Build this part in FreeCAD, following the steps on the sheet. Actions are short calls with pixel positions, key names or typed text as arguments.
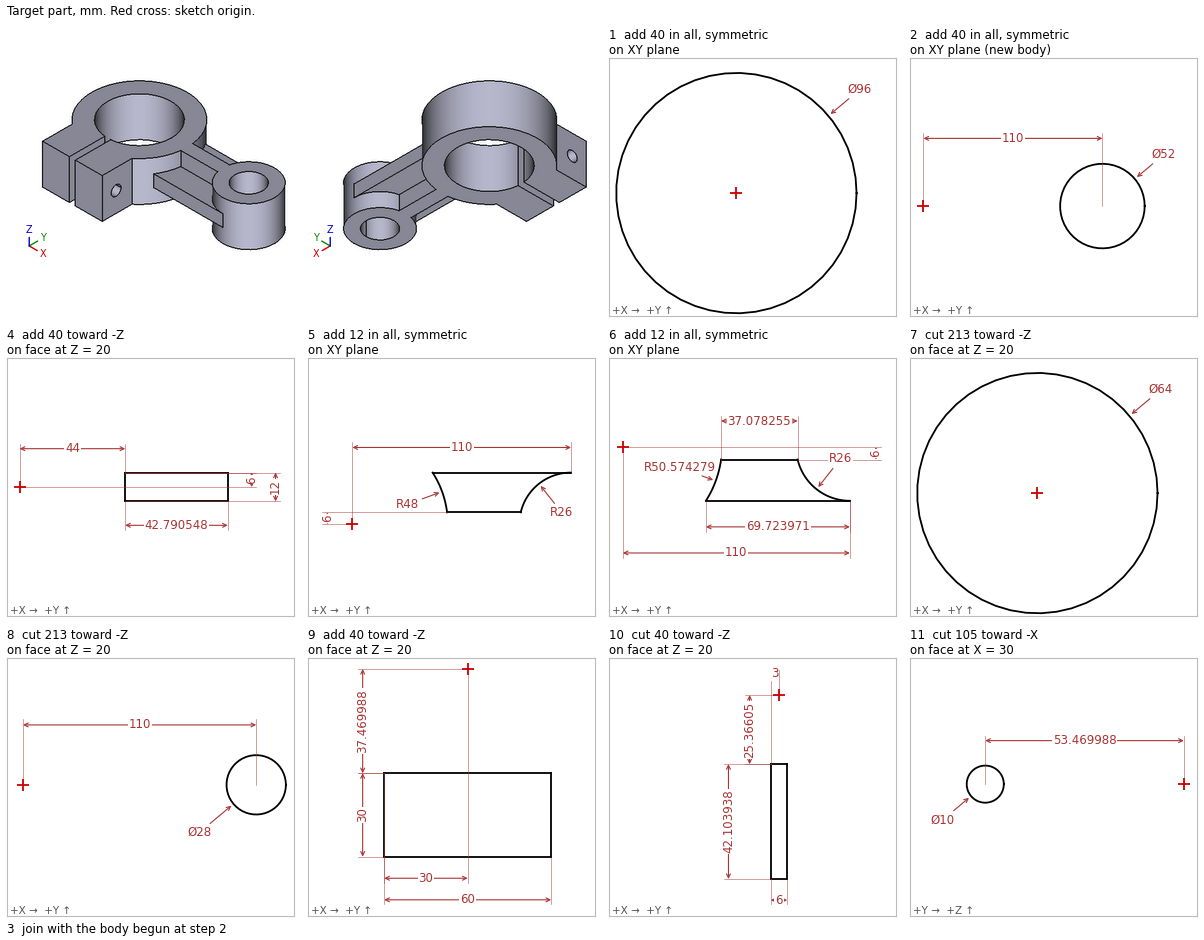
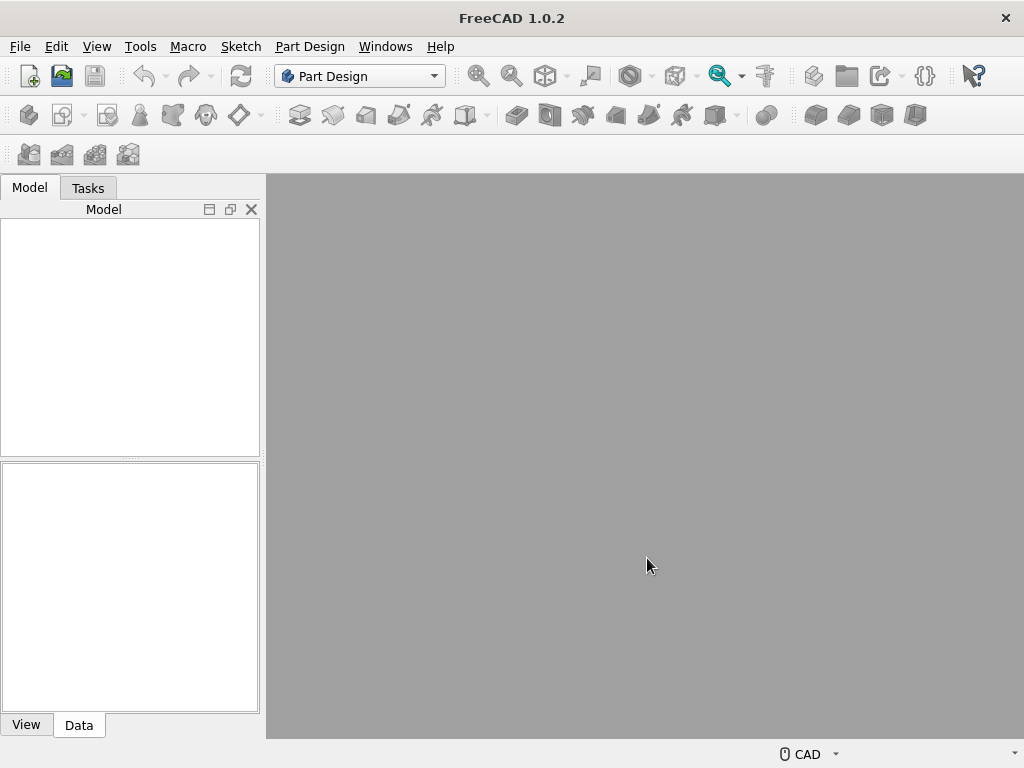
click(29, 76)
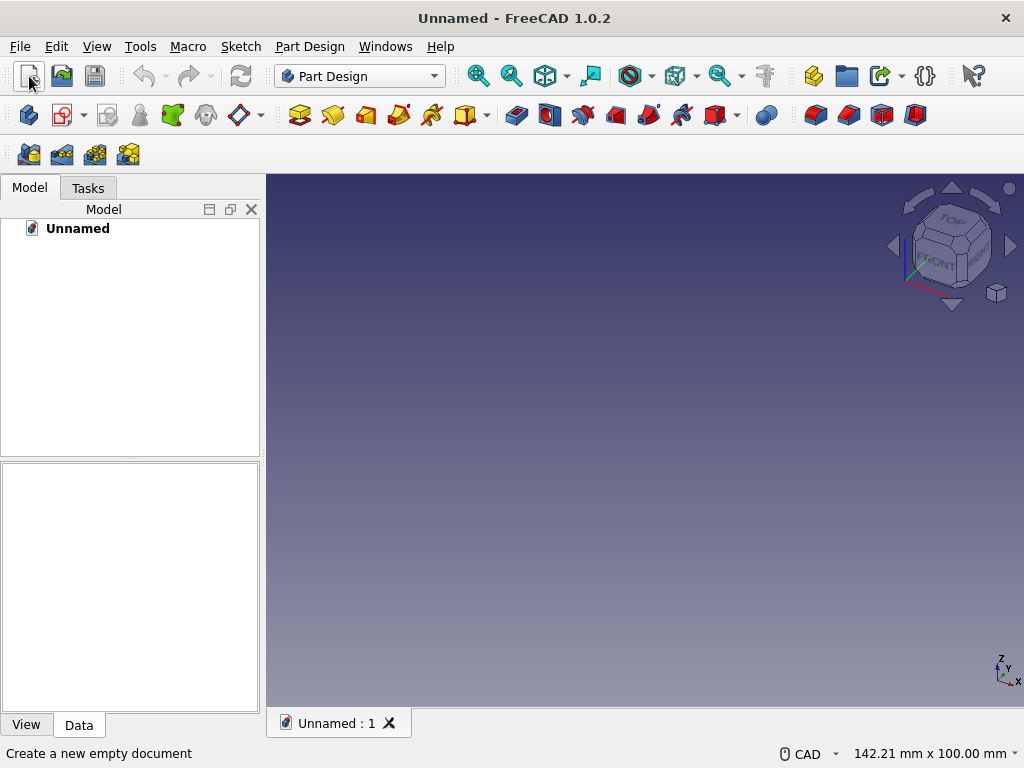
click(62, 116)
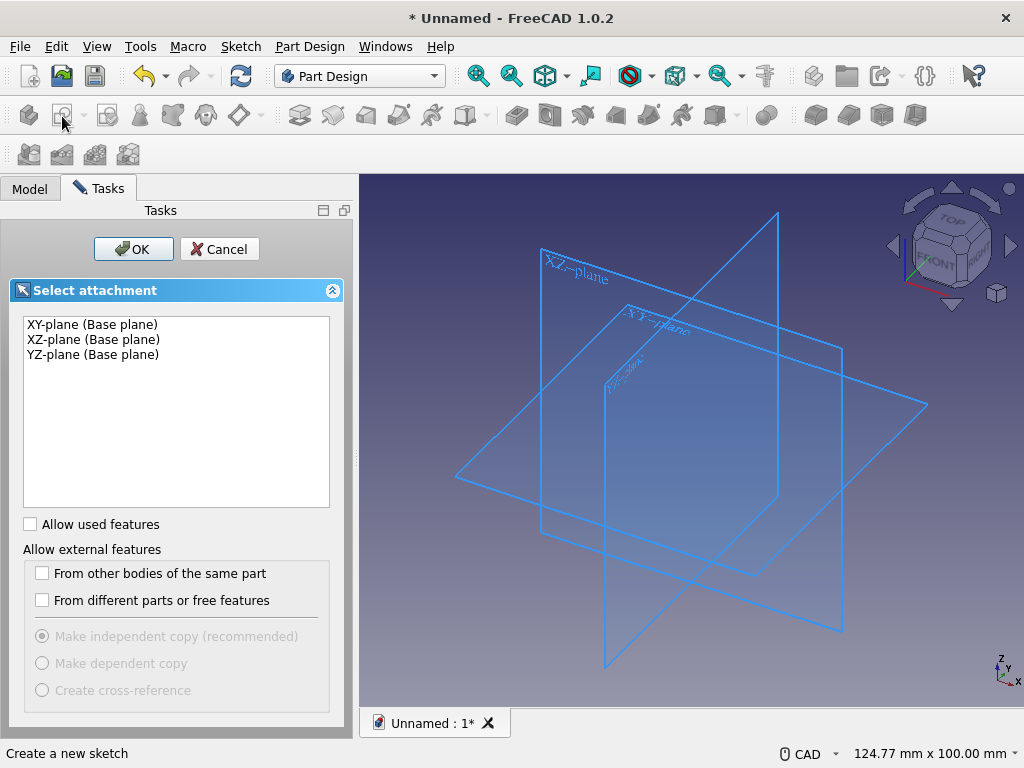
click(84, 324)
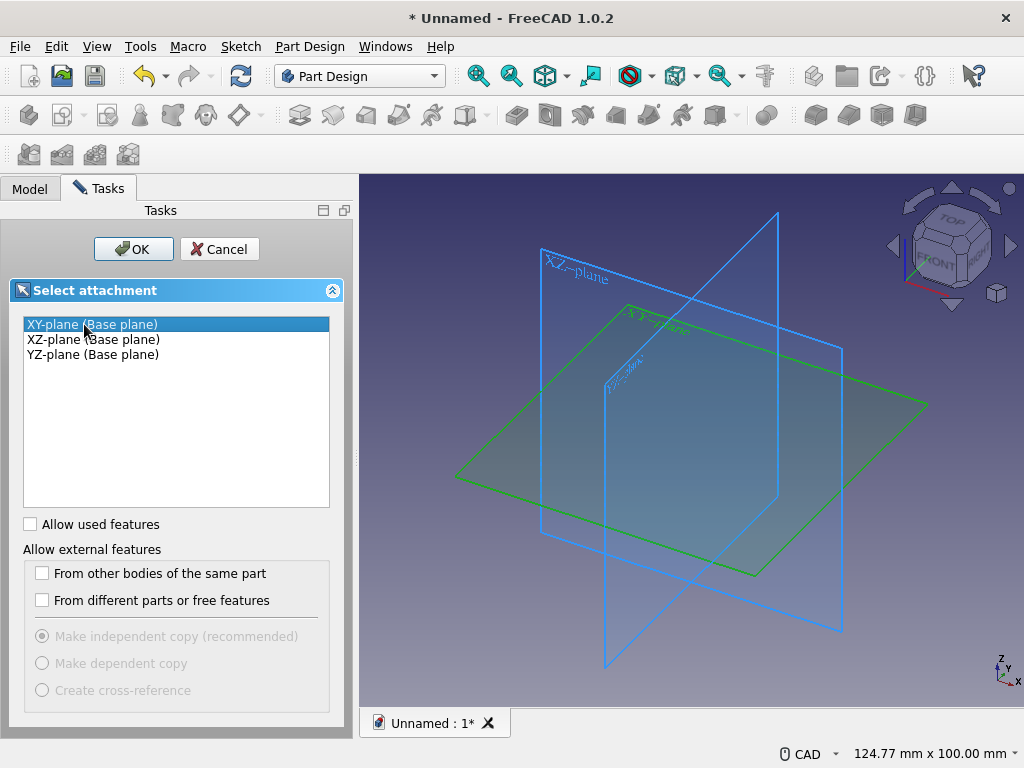
click(134, 249)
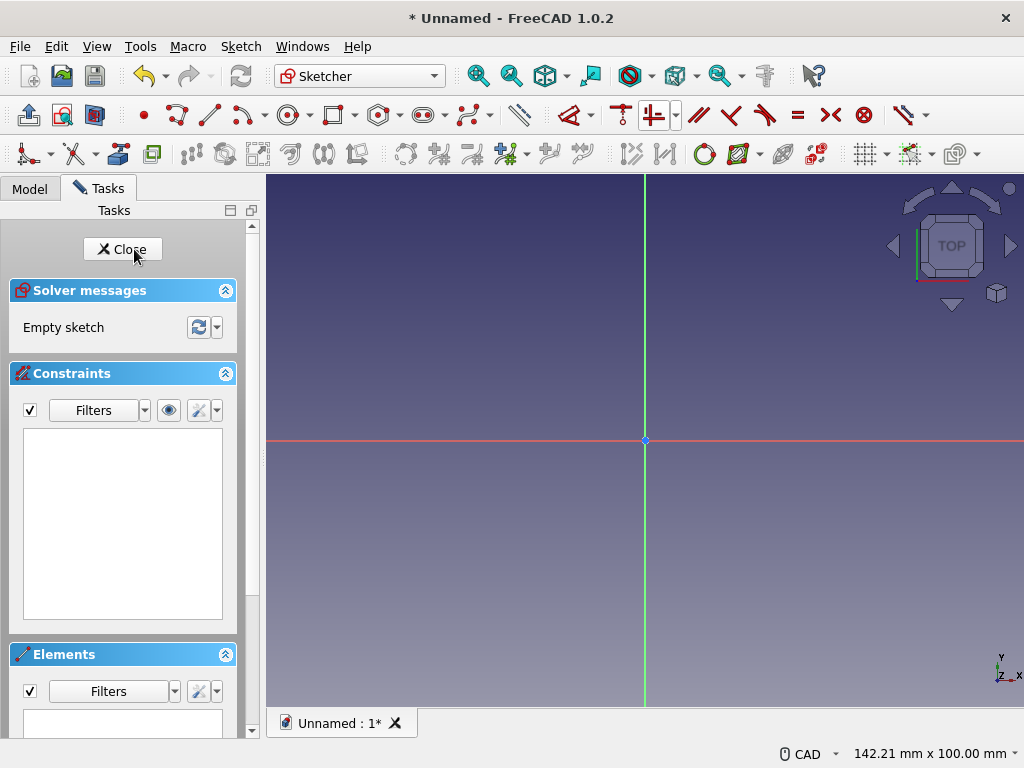
scroll(437, 440, down, 2)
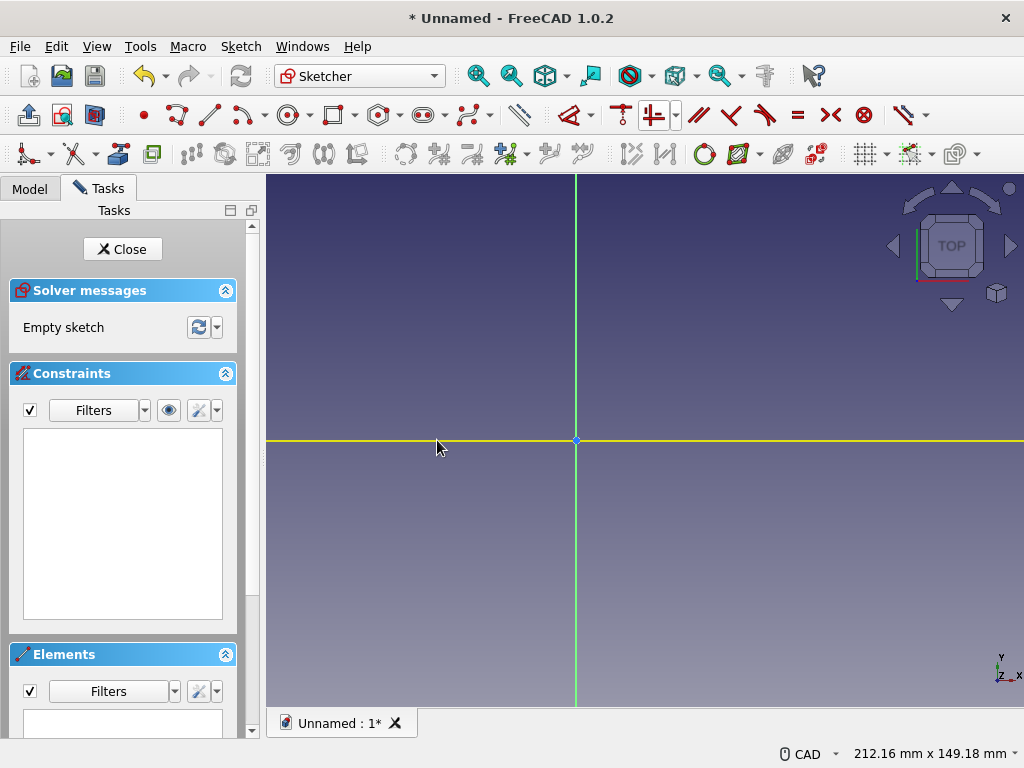
click(288, 116)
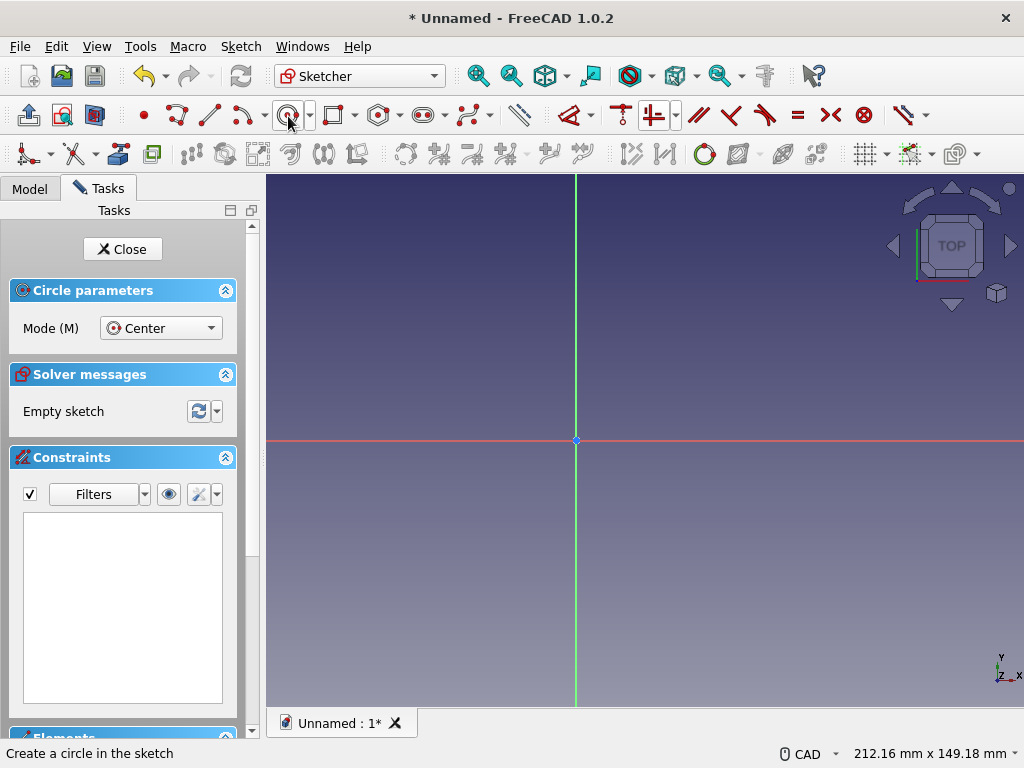
click(577, 440)
click(698, 319)
key(Escape)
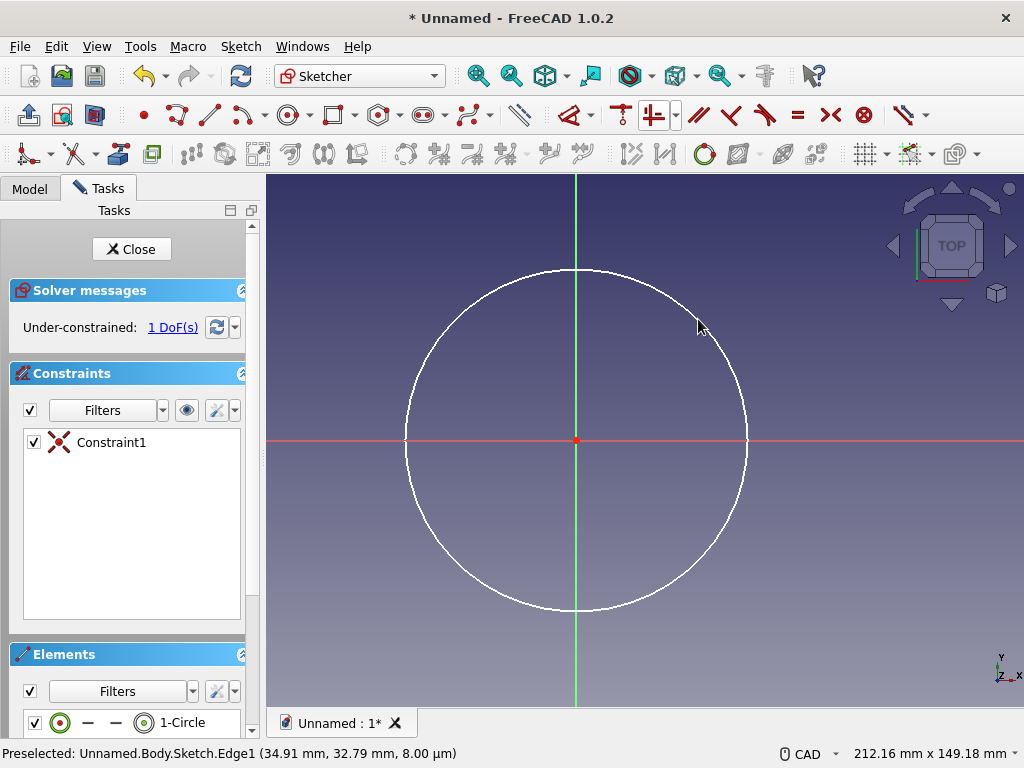
click(697, 319)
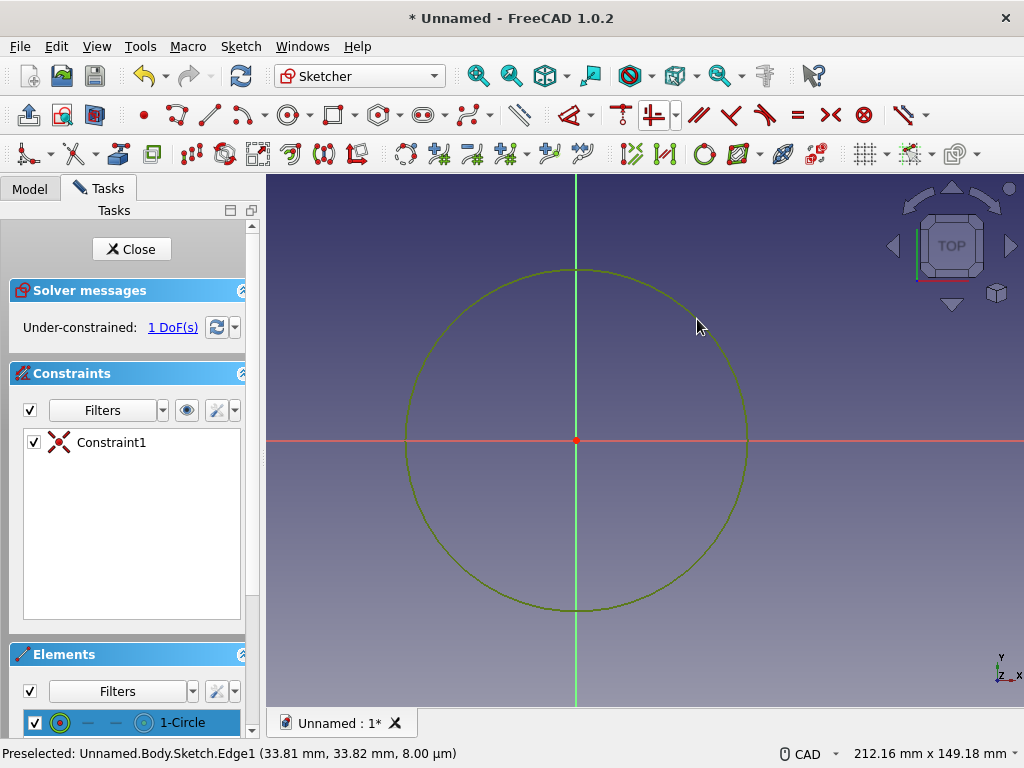
click(590, 116)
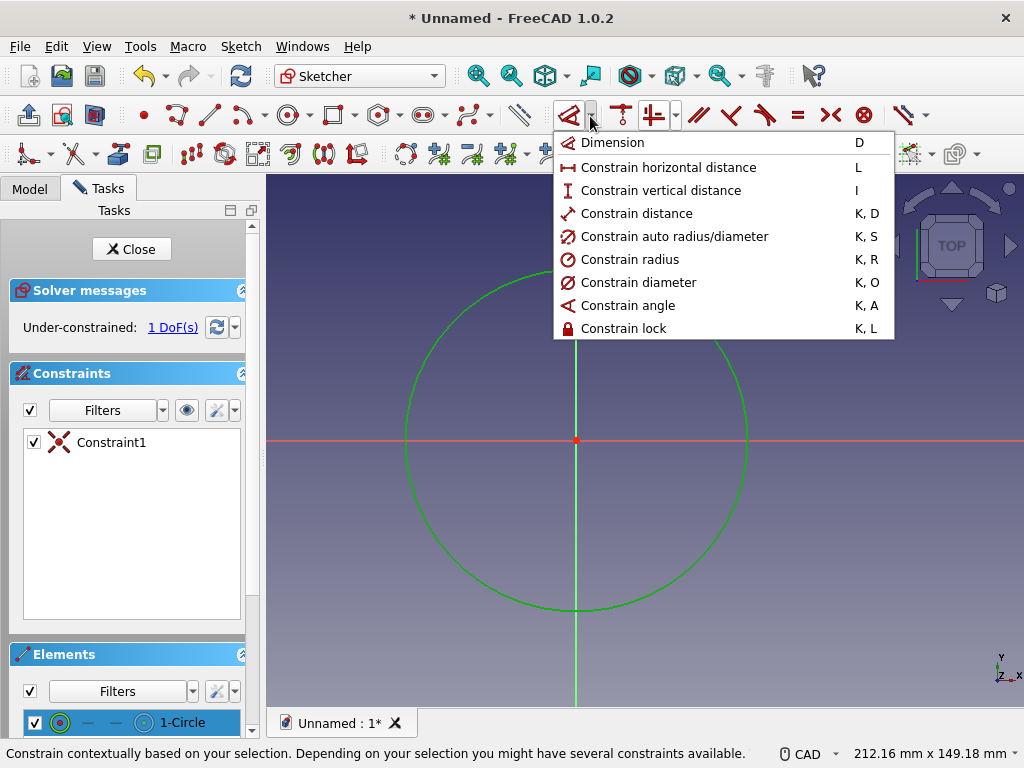
click(724, 282)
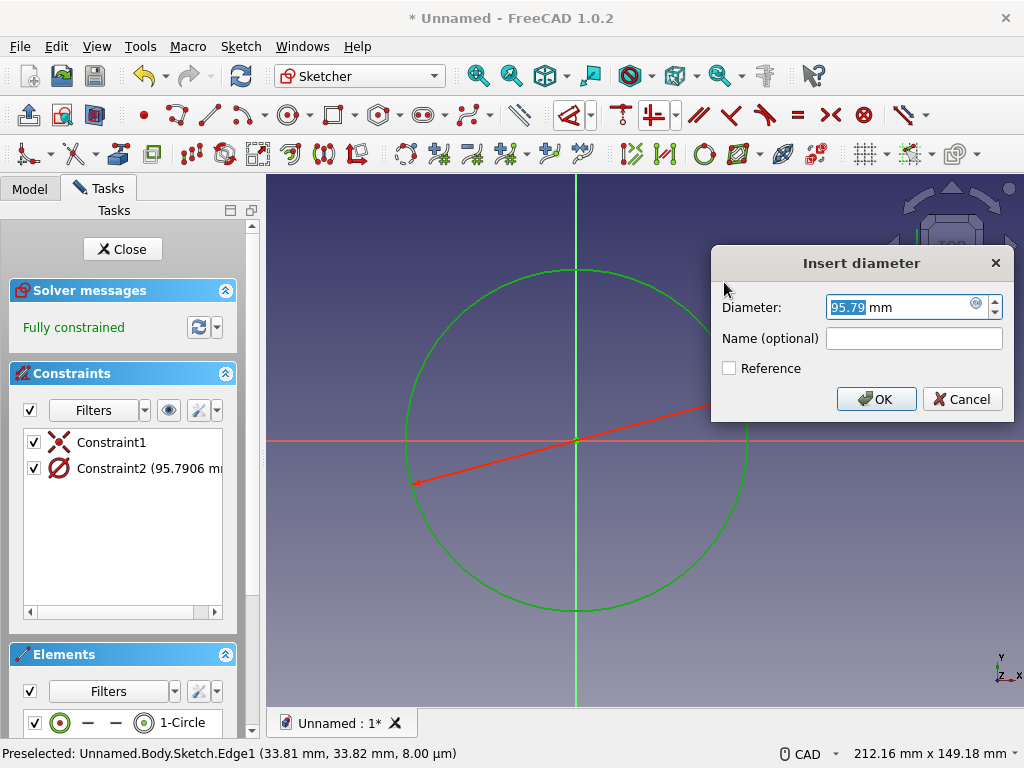
text(96)
key(Return)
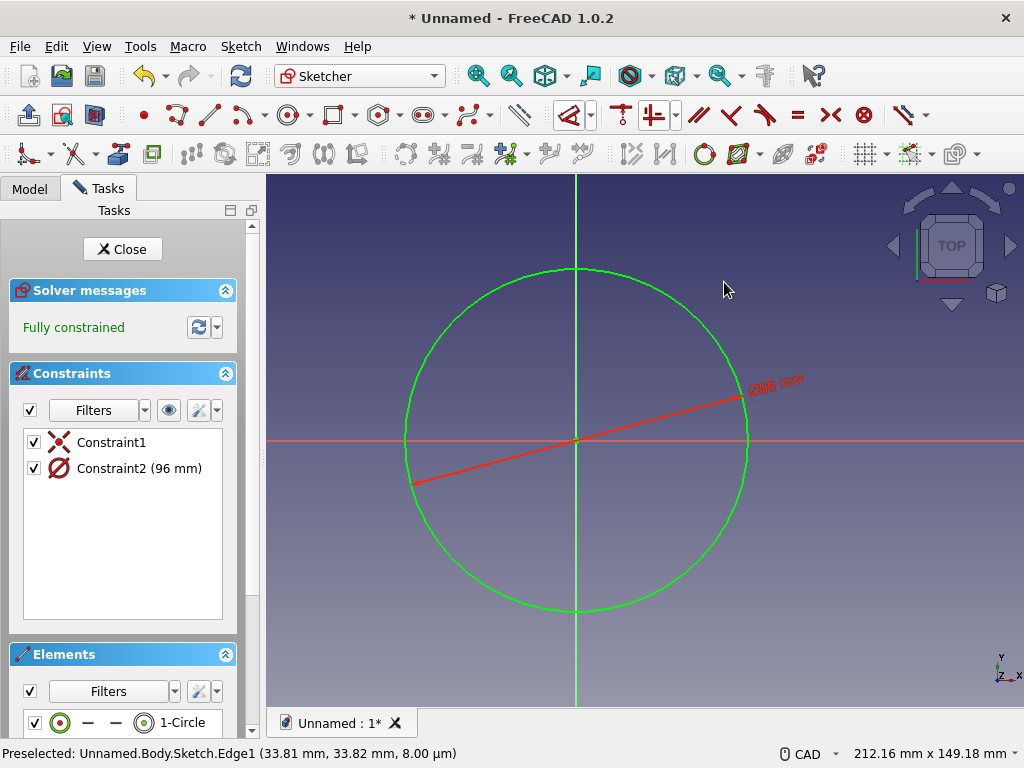
click(123, 249)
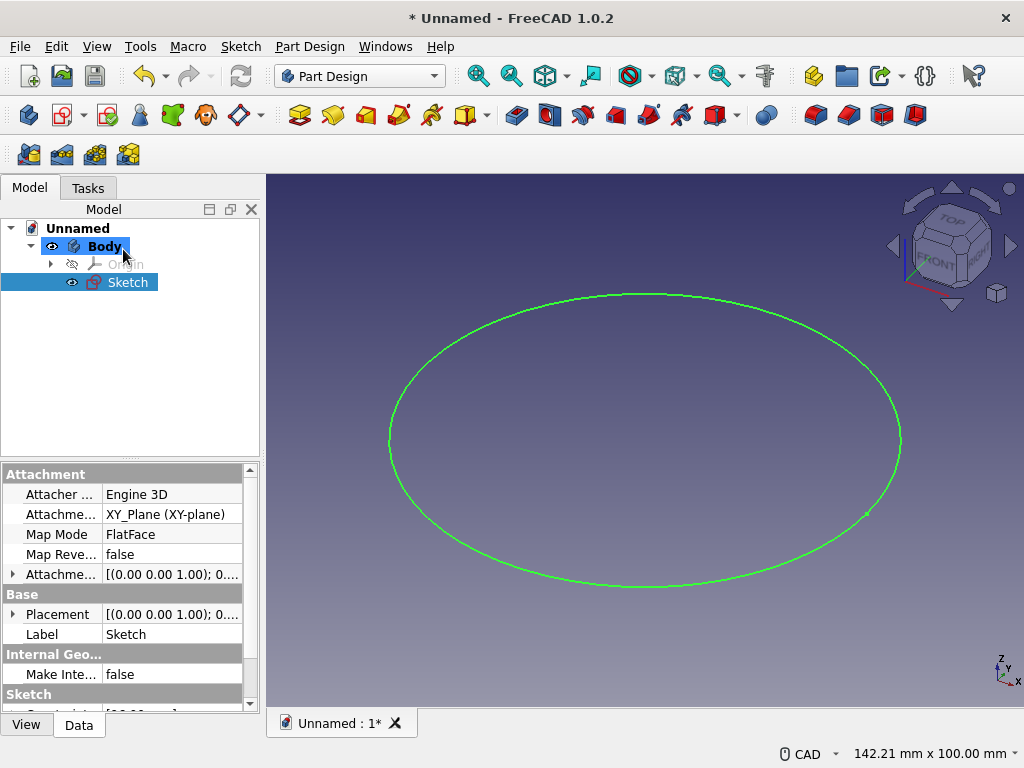
click(300, 116)